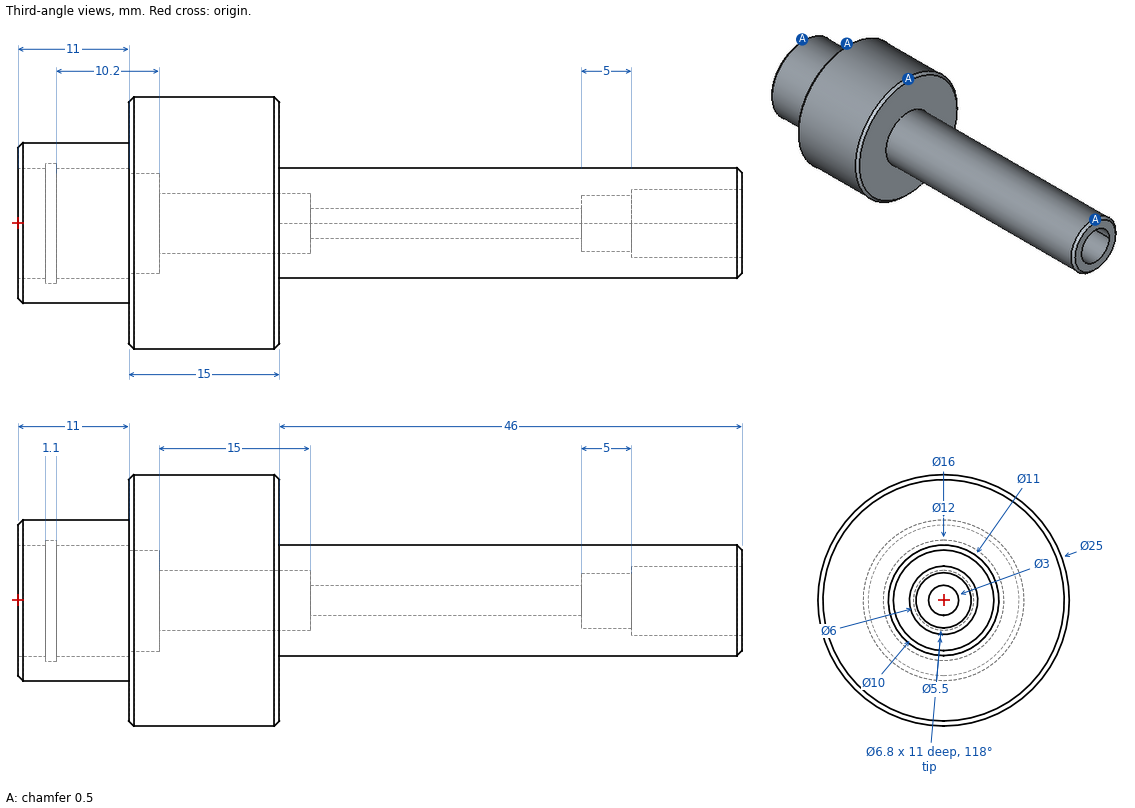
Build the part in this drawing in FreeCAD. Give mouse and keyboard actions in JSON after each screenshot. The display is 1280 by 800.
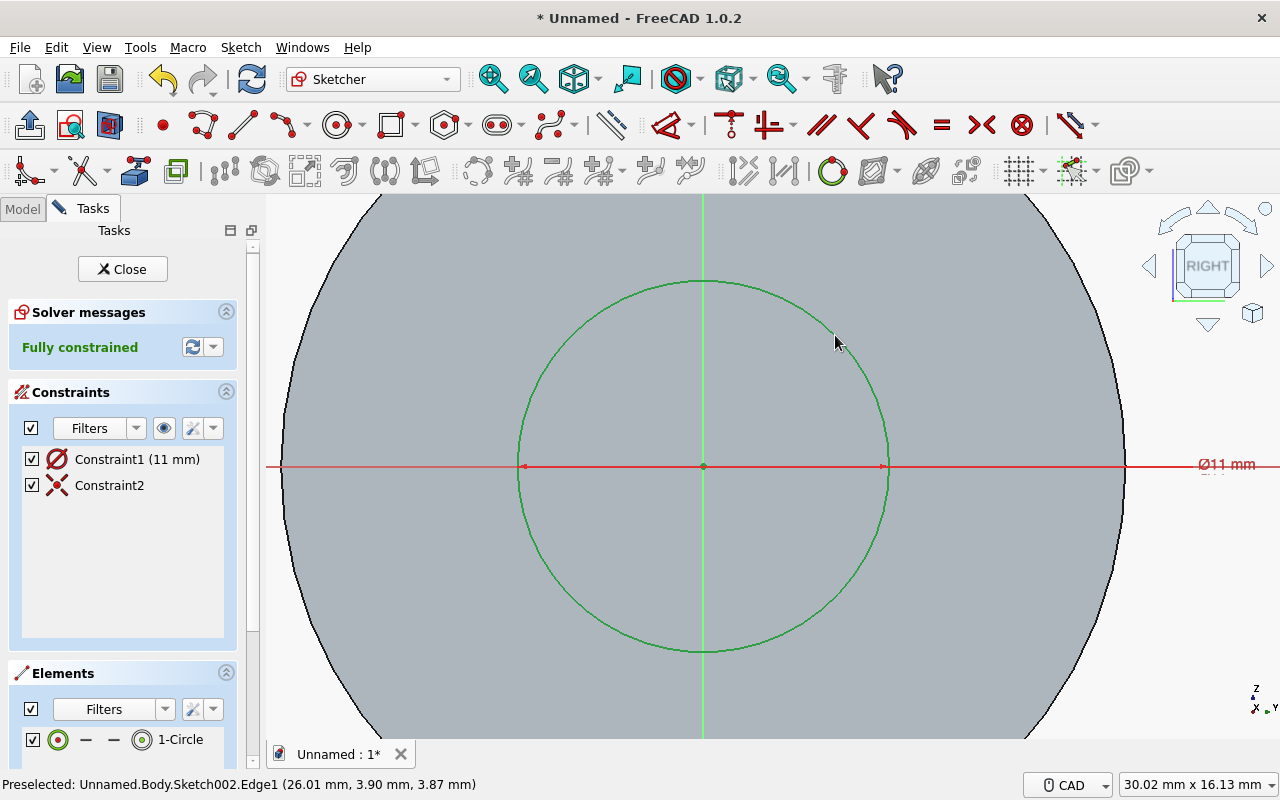
{"action": "left_click", "coordinate": [123, 269]}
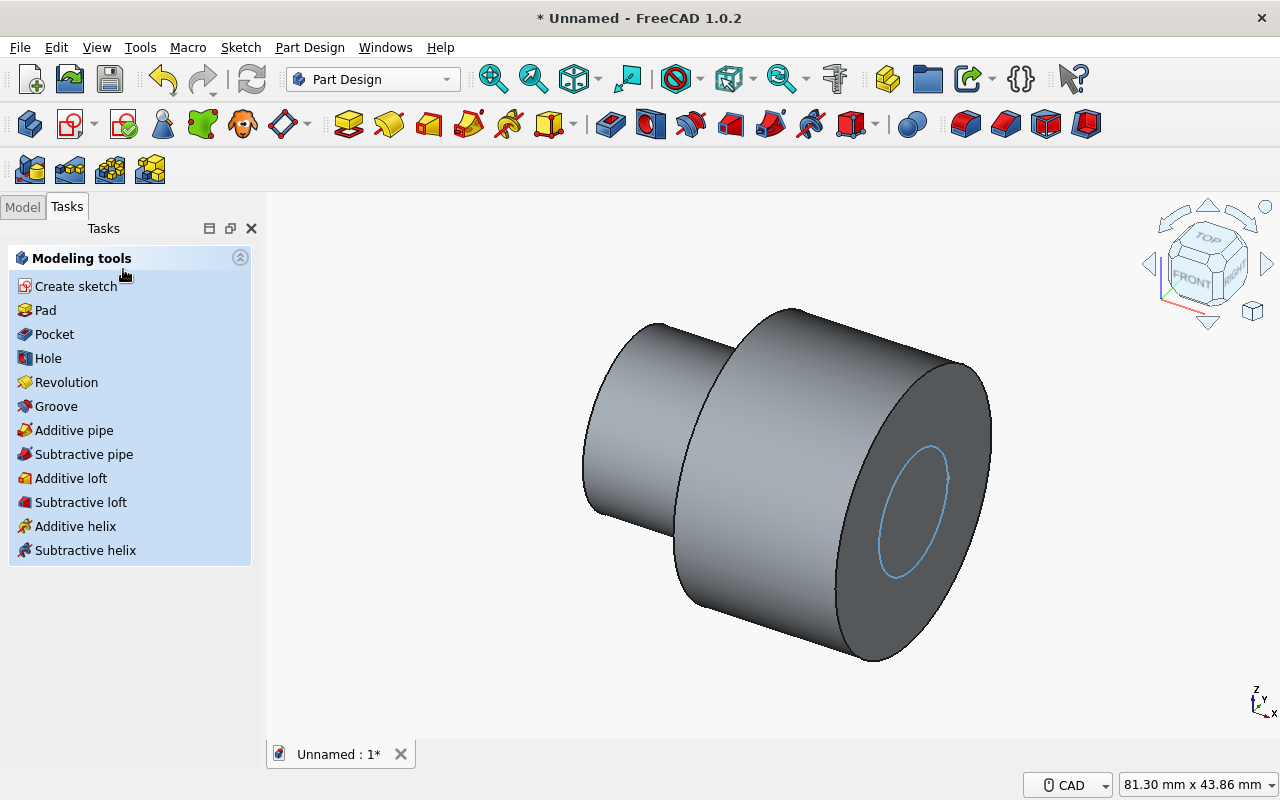
{"action": "left_click", "coordinate": [350, 124]}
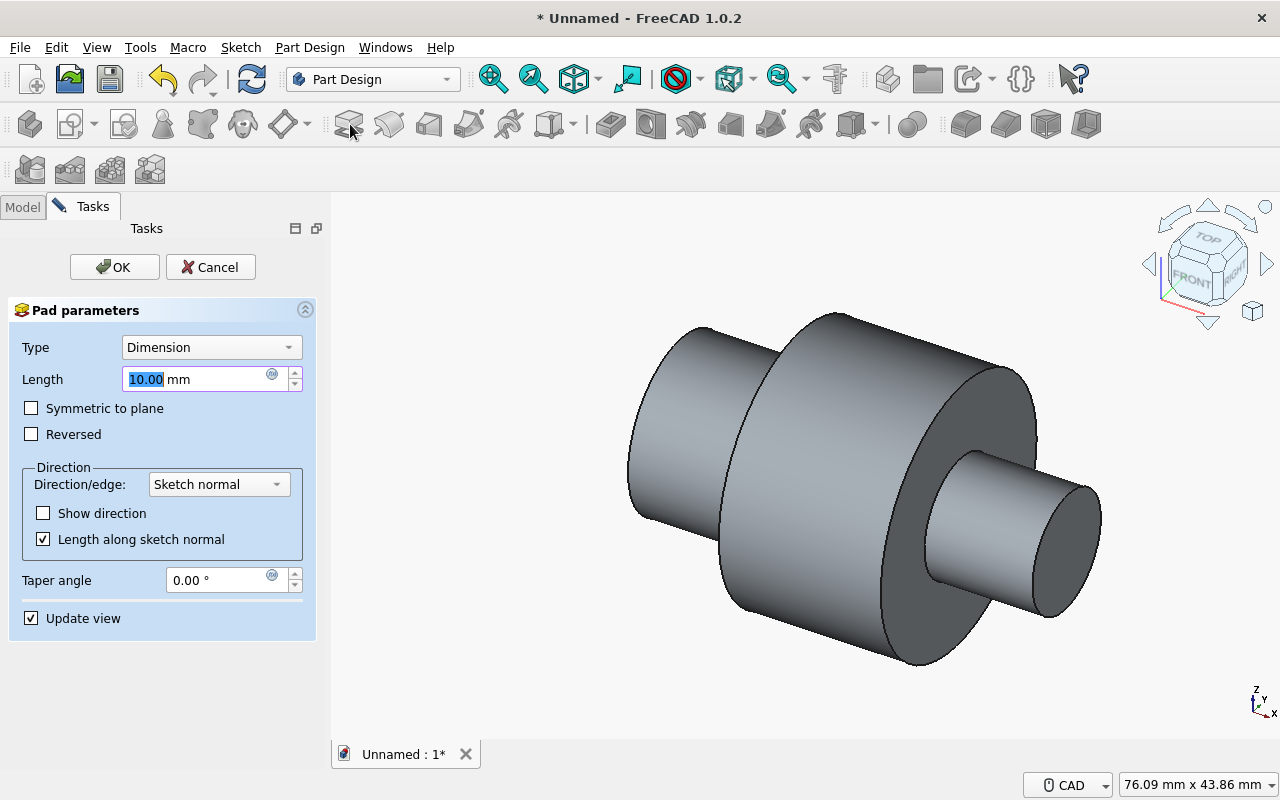
{"action": "type", "text": "46"}
{"action": "key", "text": "Tab"}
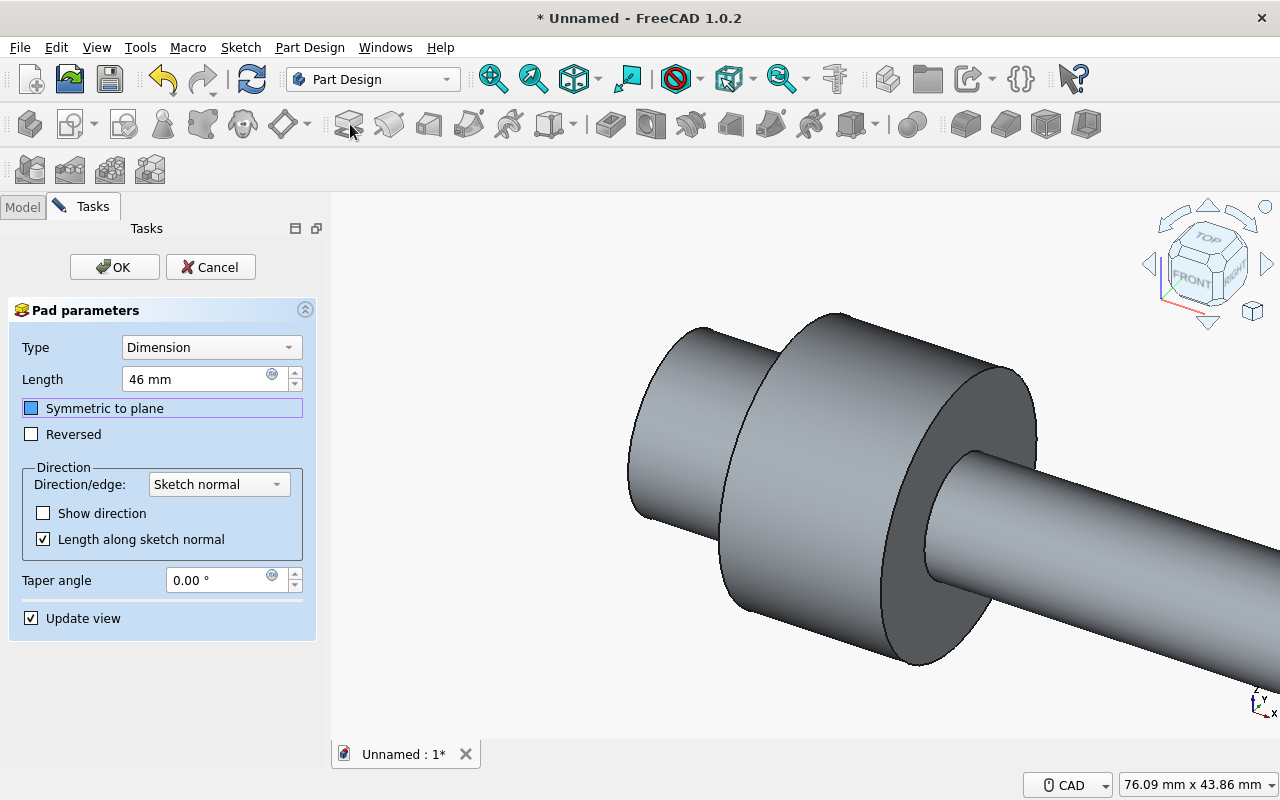
{"action": "left_click", "coordinate": [115, 267]}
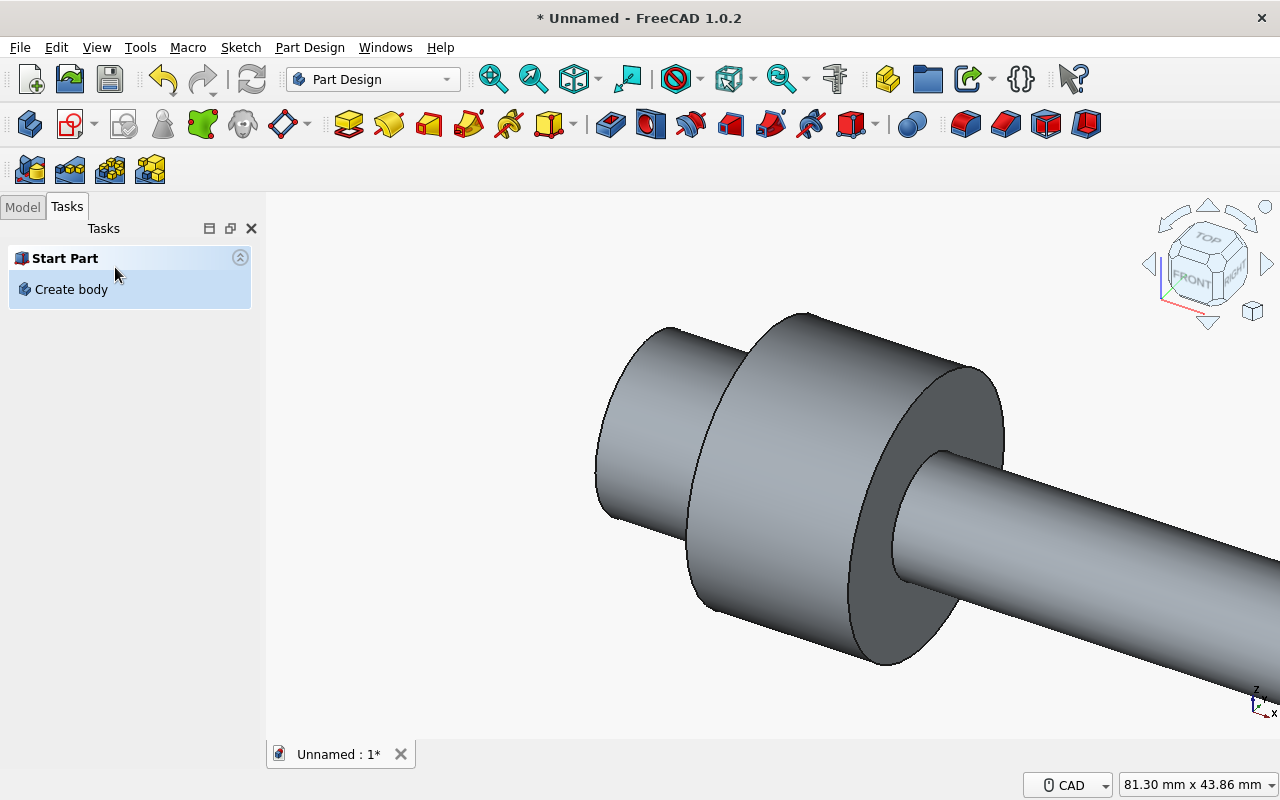
{"action": "left_click", "coordinate": [494, 80]}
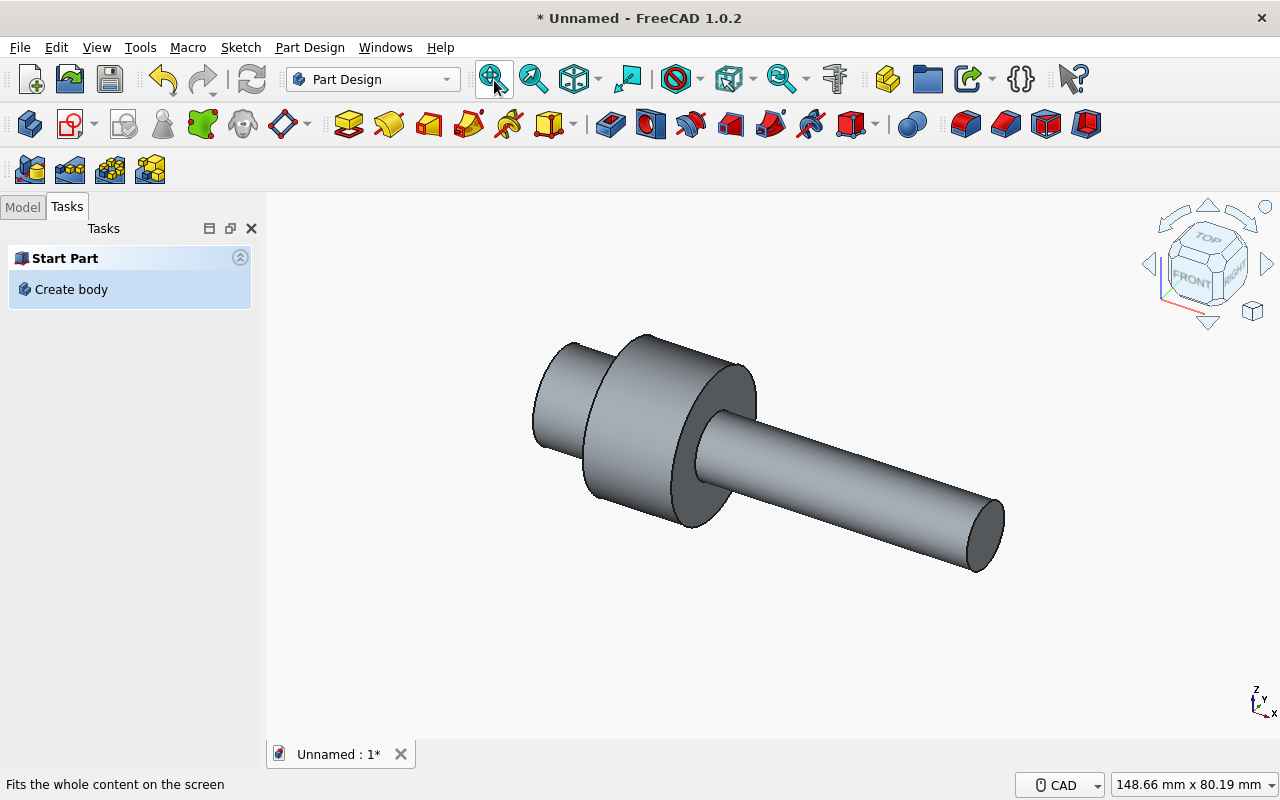
{"action": "key", "text": "6"}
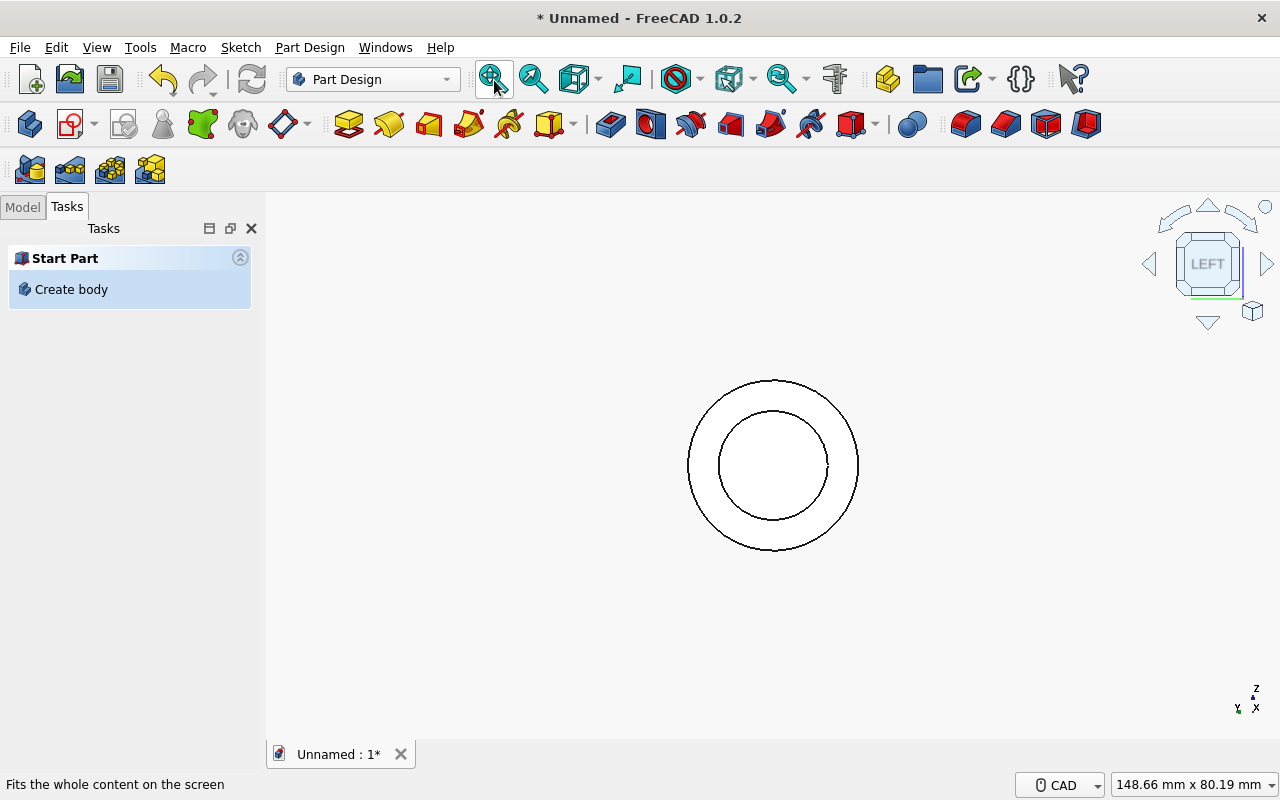
{"action": "left_click", "coordinate": [494, 80]}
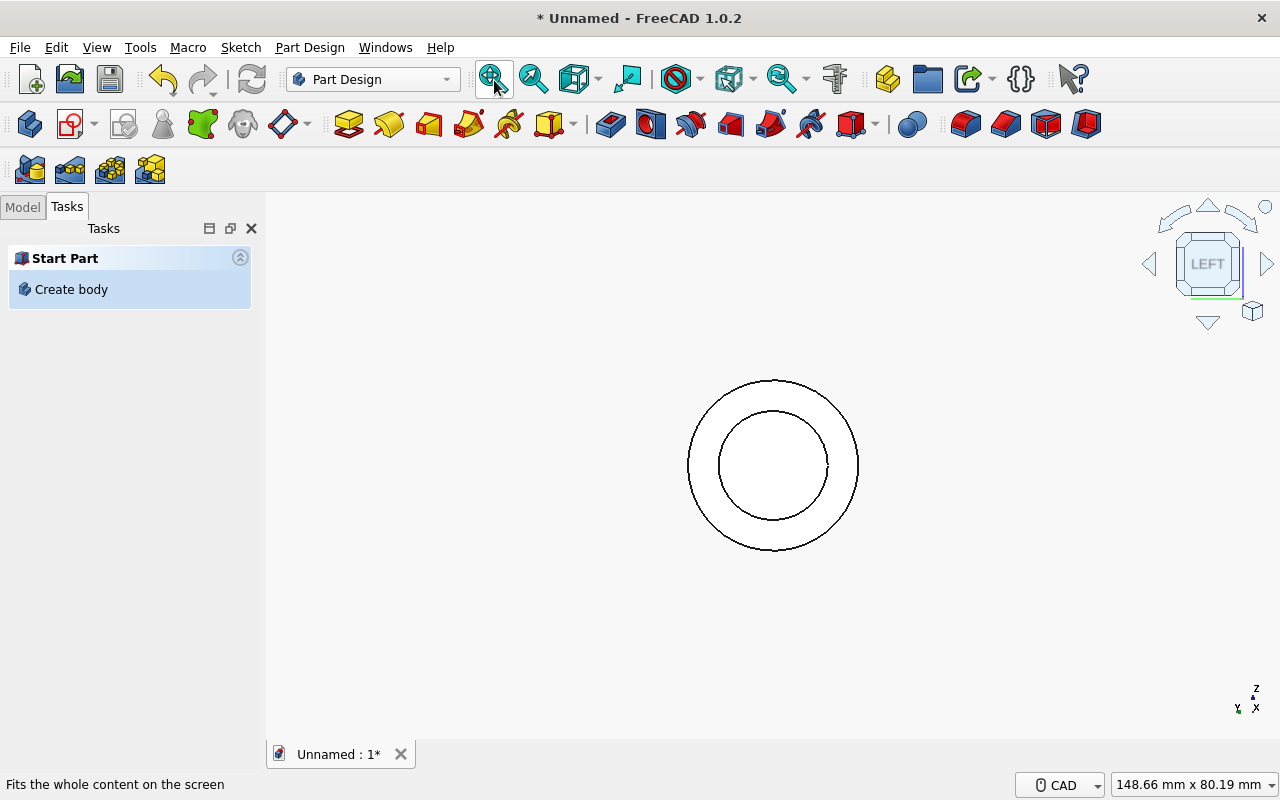
{"action": "left_click", "coordinate": [773, 464]}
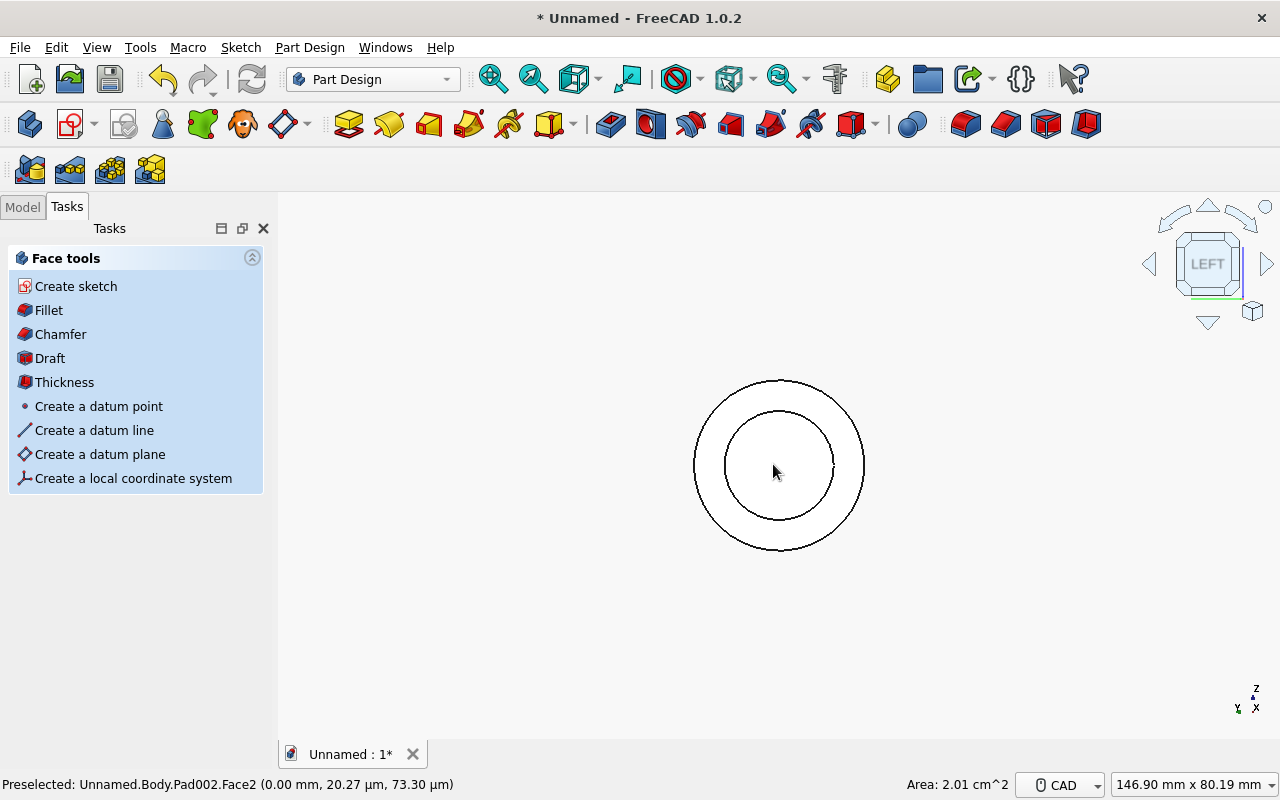
{"action": "left_click", "coordinate": [70, 124]}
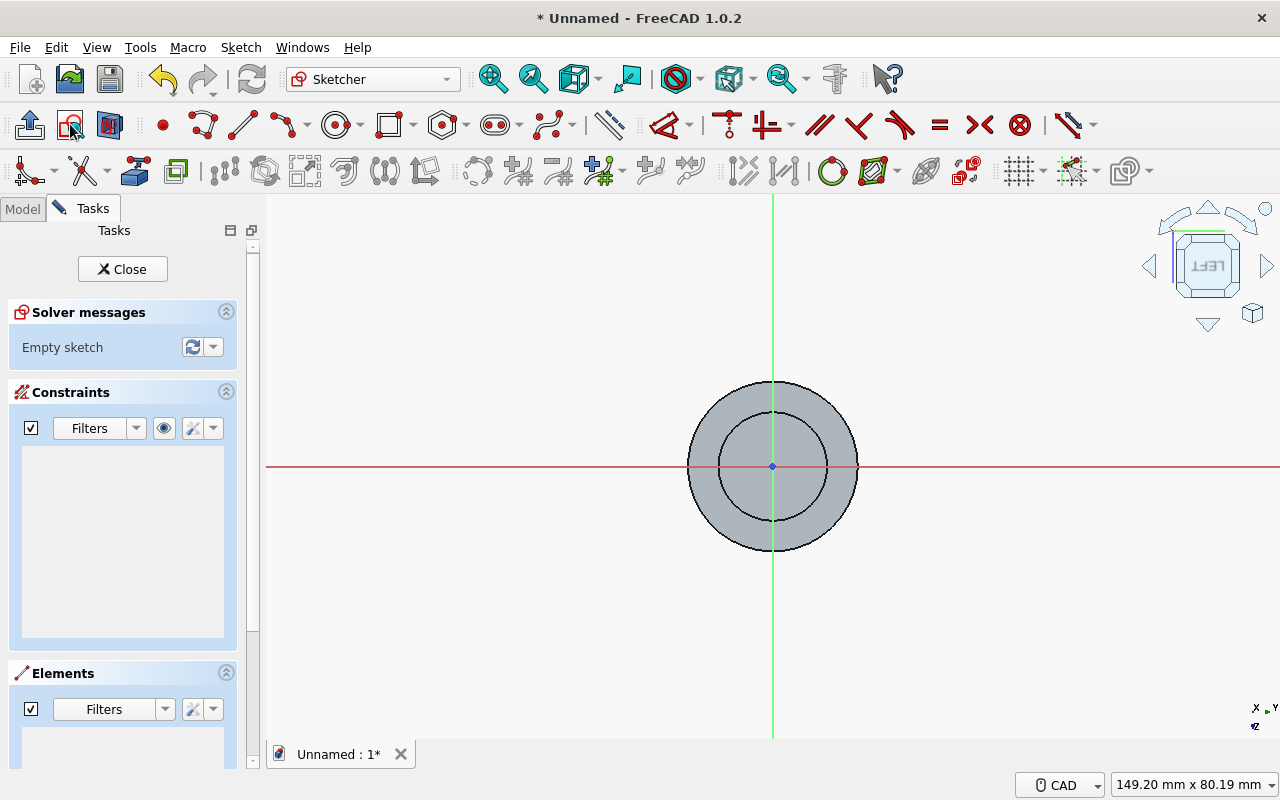
{"action": "scroll", "coordinate": [790, 466], "scroll_direction": "up", "scroll_amount": 8}